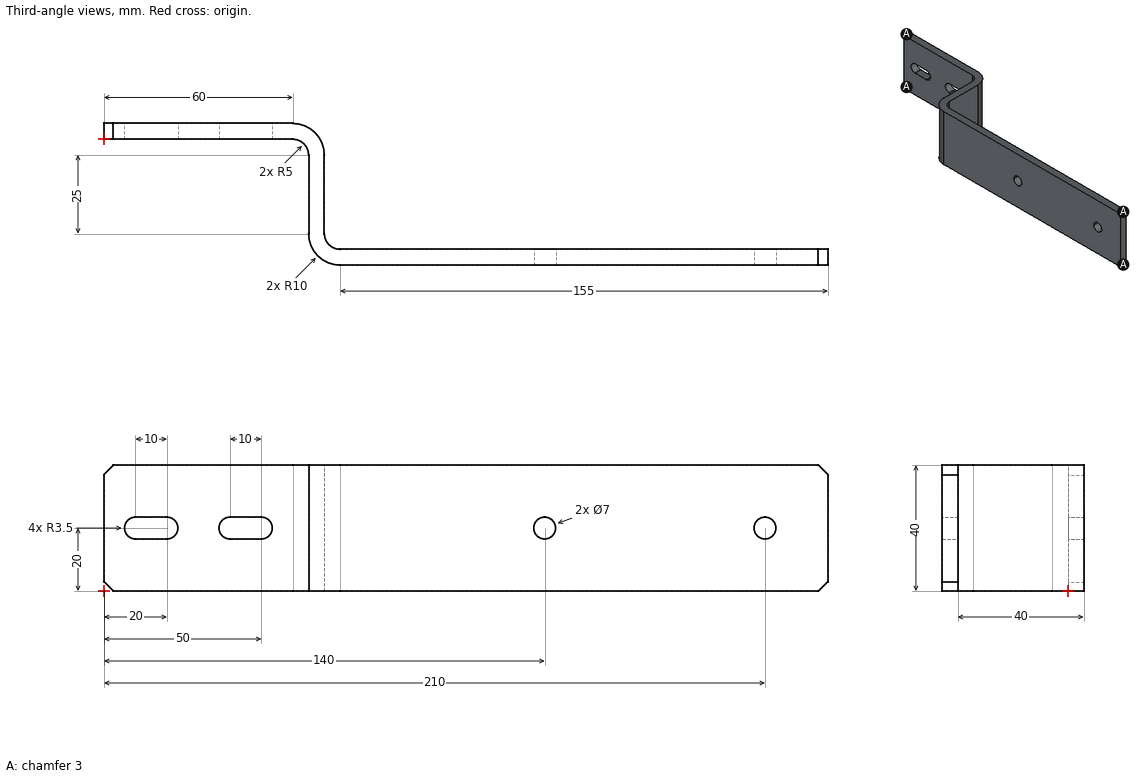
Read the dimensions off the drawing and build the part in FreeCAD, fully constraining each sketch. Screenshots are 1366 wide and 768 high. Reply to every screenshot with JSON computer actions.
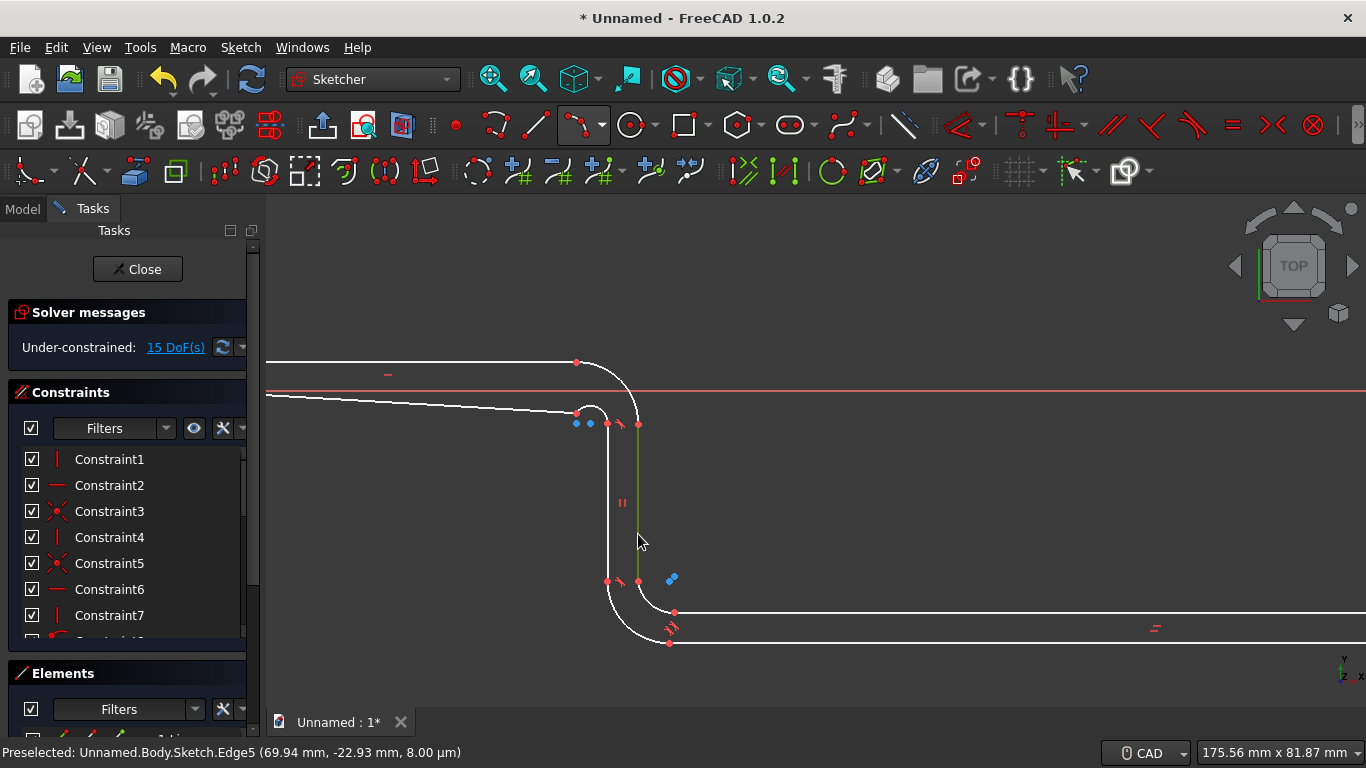
{"action": "left_click", "coordinate": [644, 596]}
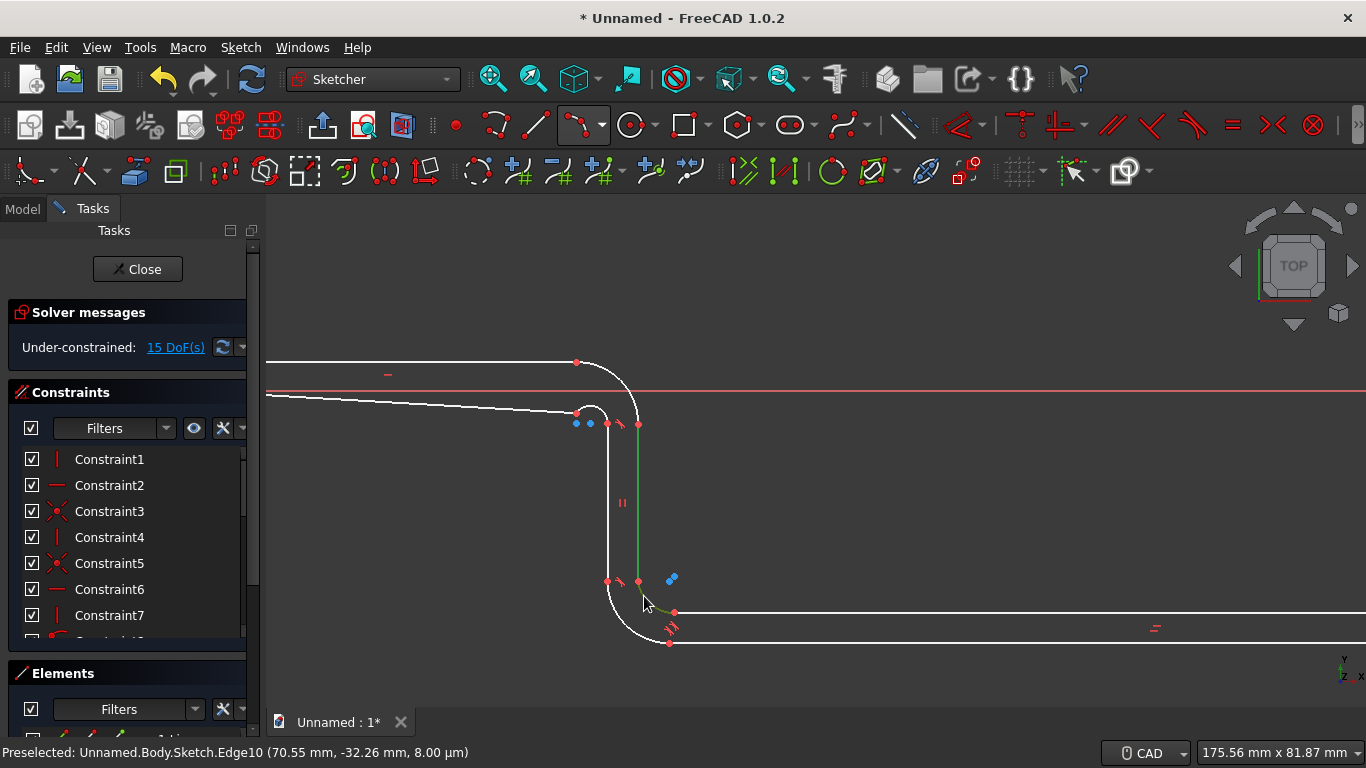
{"action": "left_click", "coordinate": [1194, 126]}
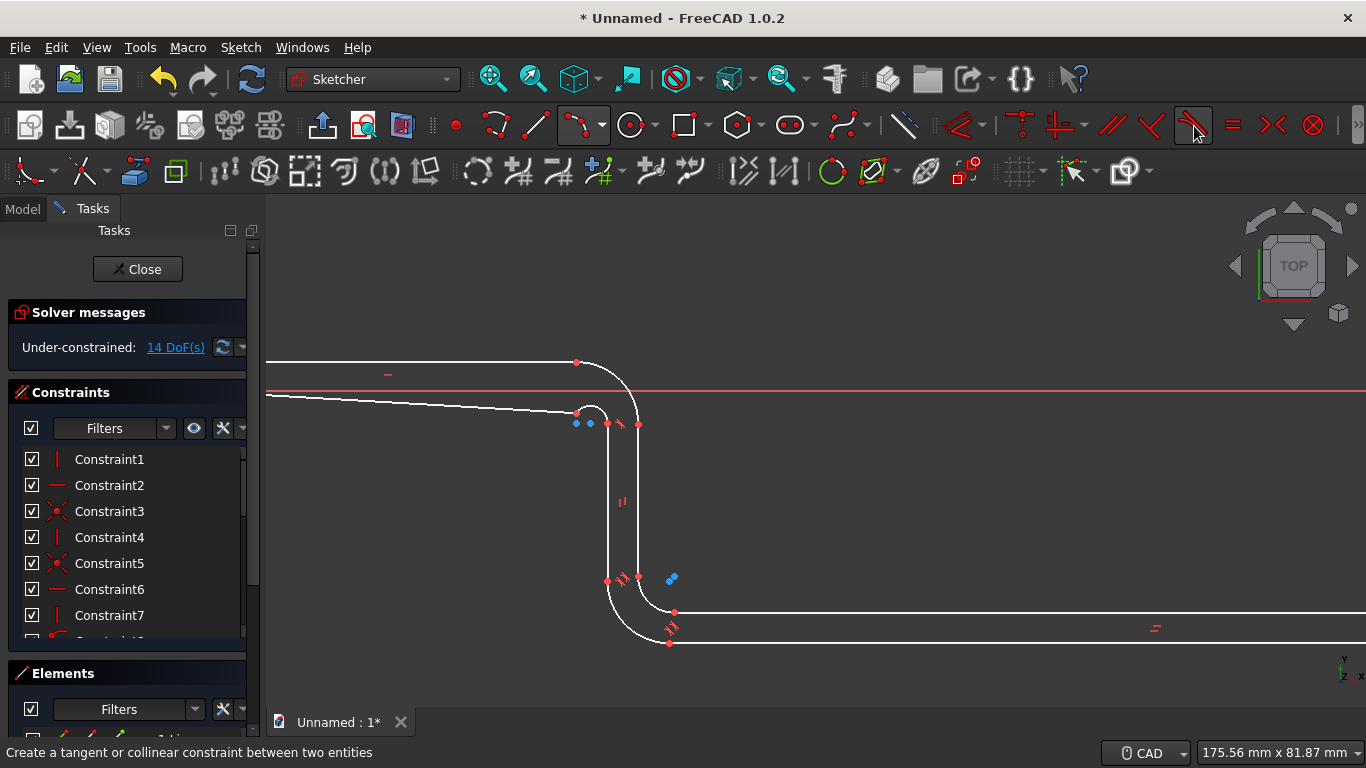
{"action": "left_click", "coordinate": [638, 531]}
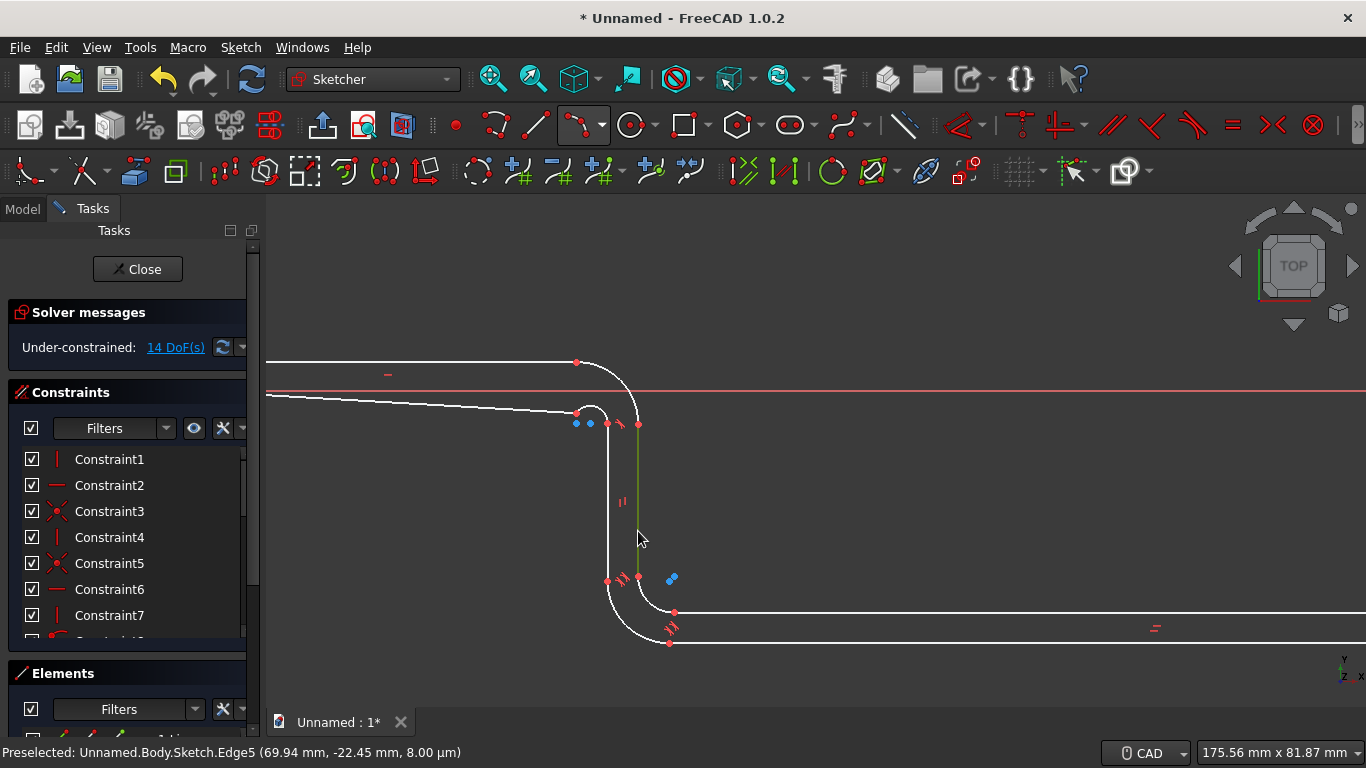
{"action": "left_click", "coordinate": [604, 369]}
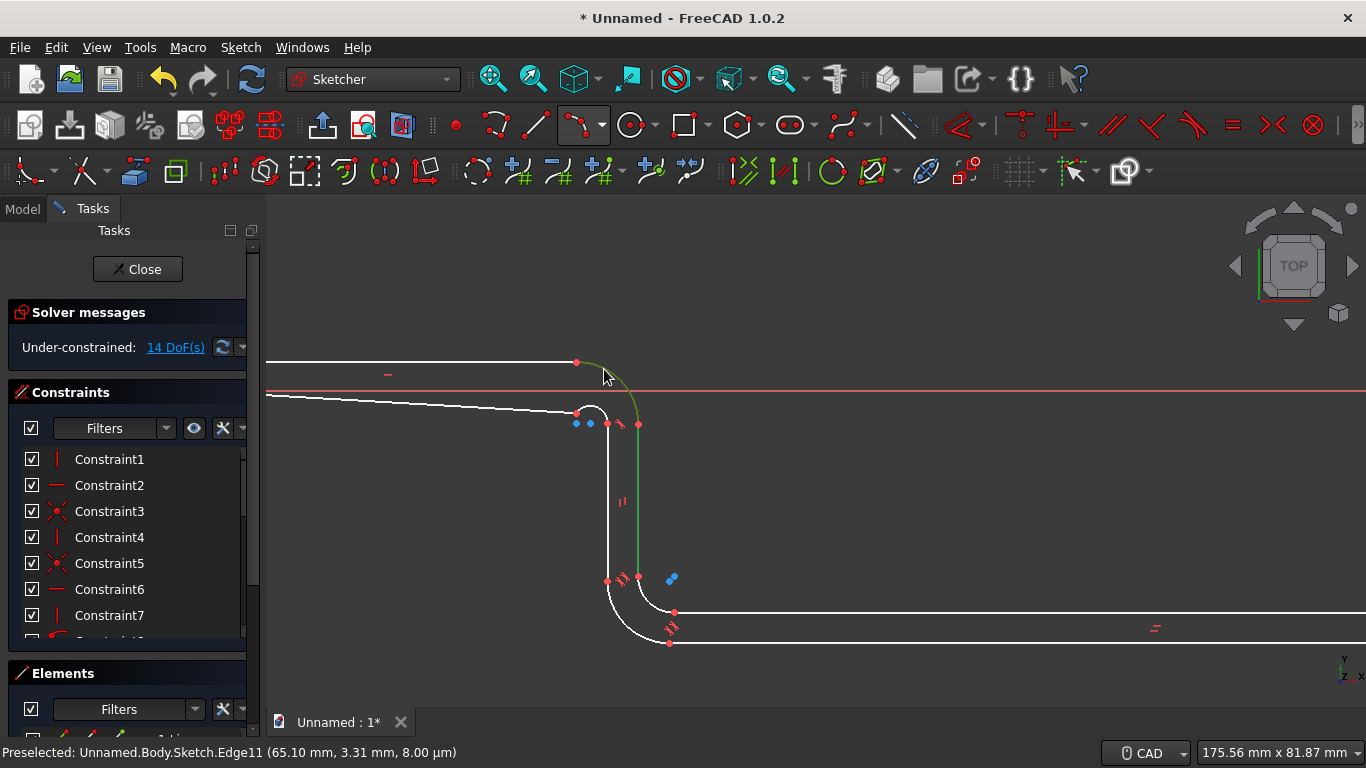
{"action": "left_click", "coordinate": [1194, 126]}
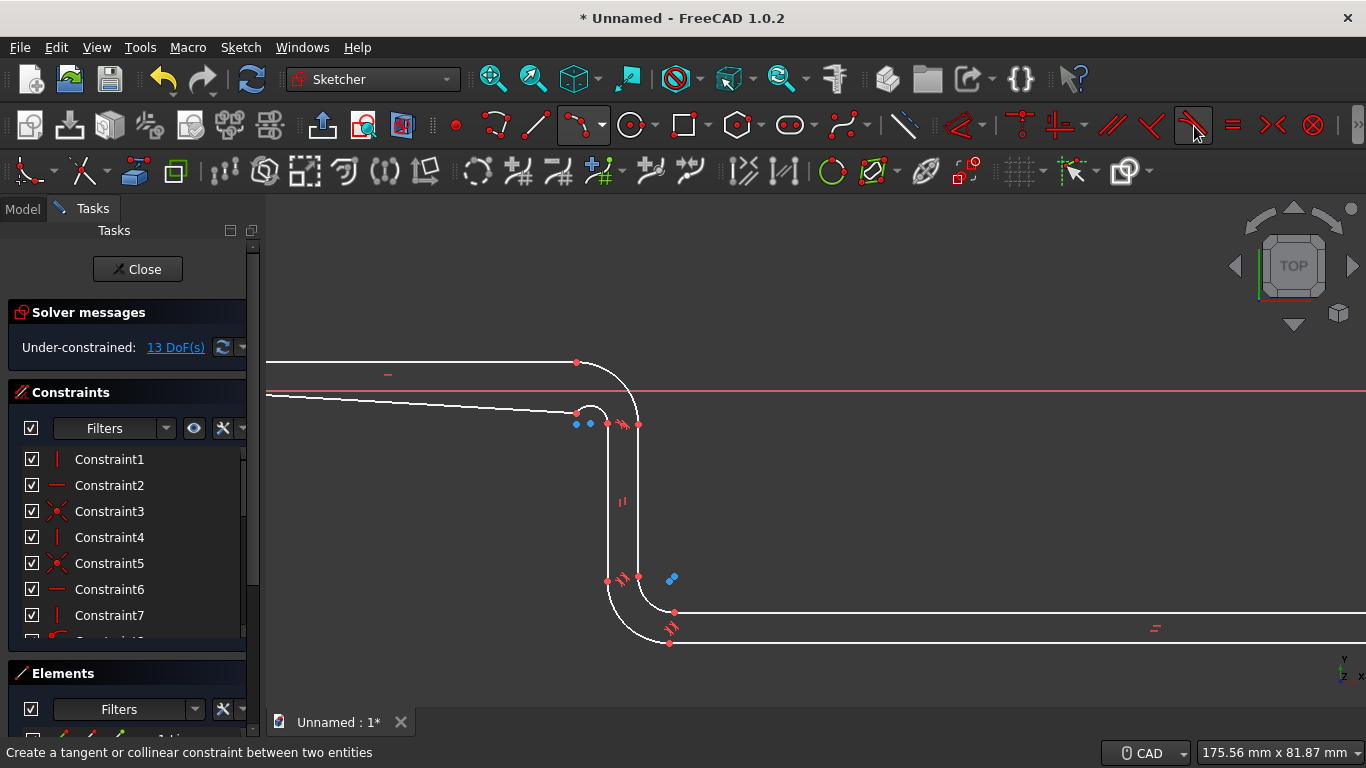
{"action": "left_click", "coordinate": [463, 362]}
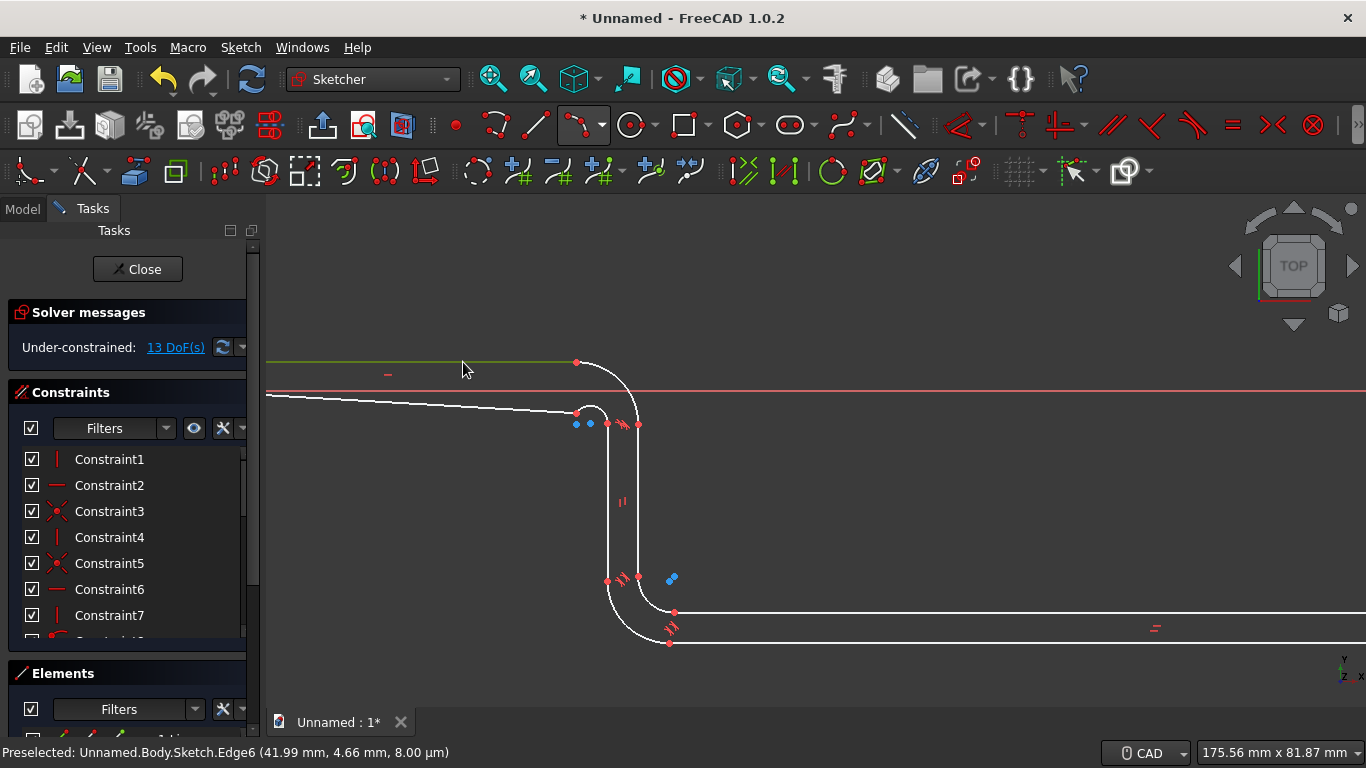
{"action": "left_click", "coordinate": [604, 369]}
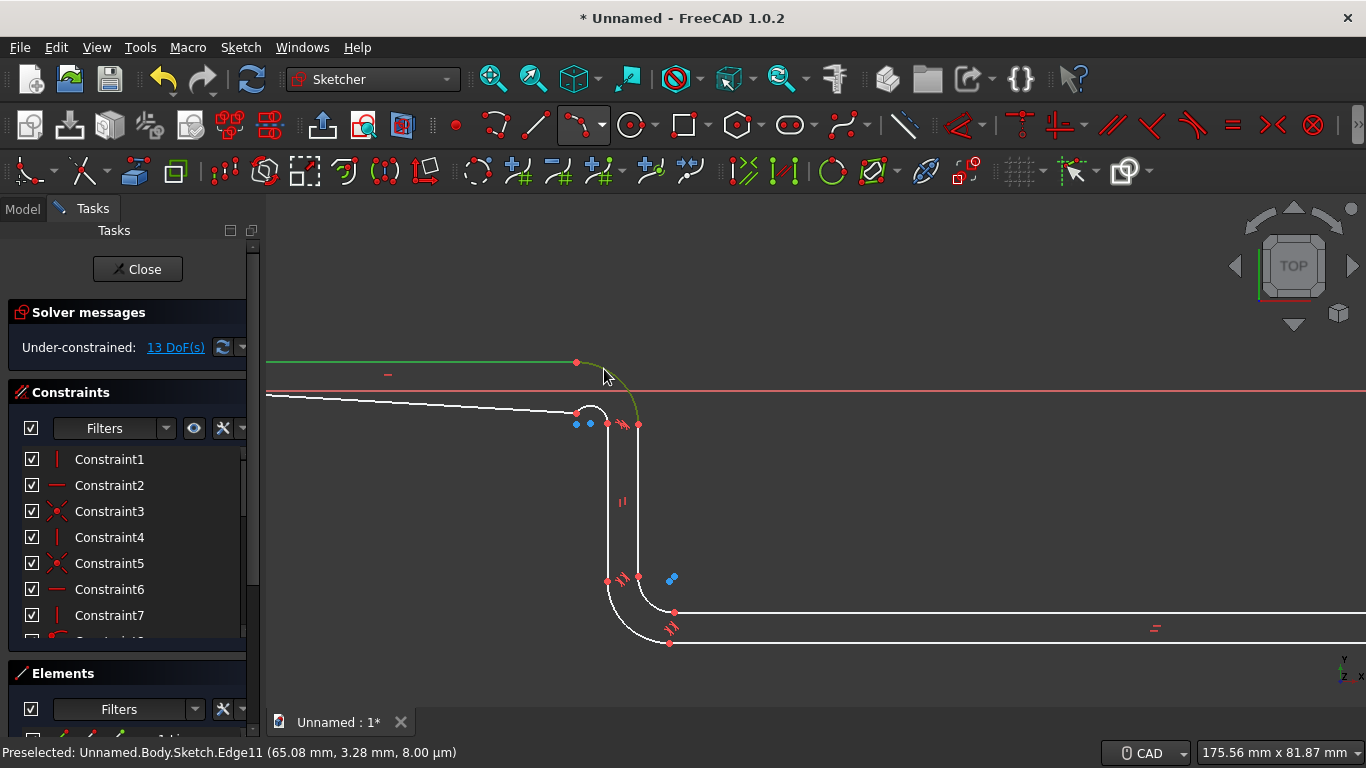
{"action": "left_click", "coordinate": [1194, 126]}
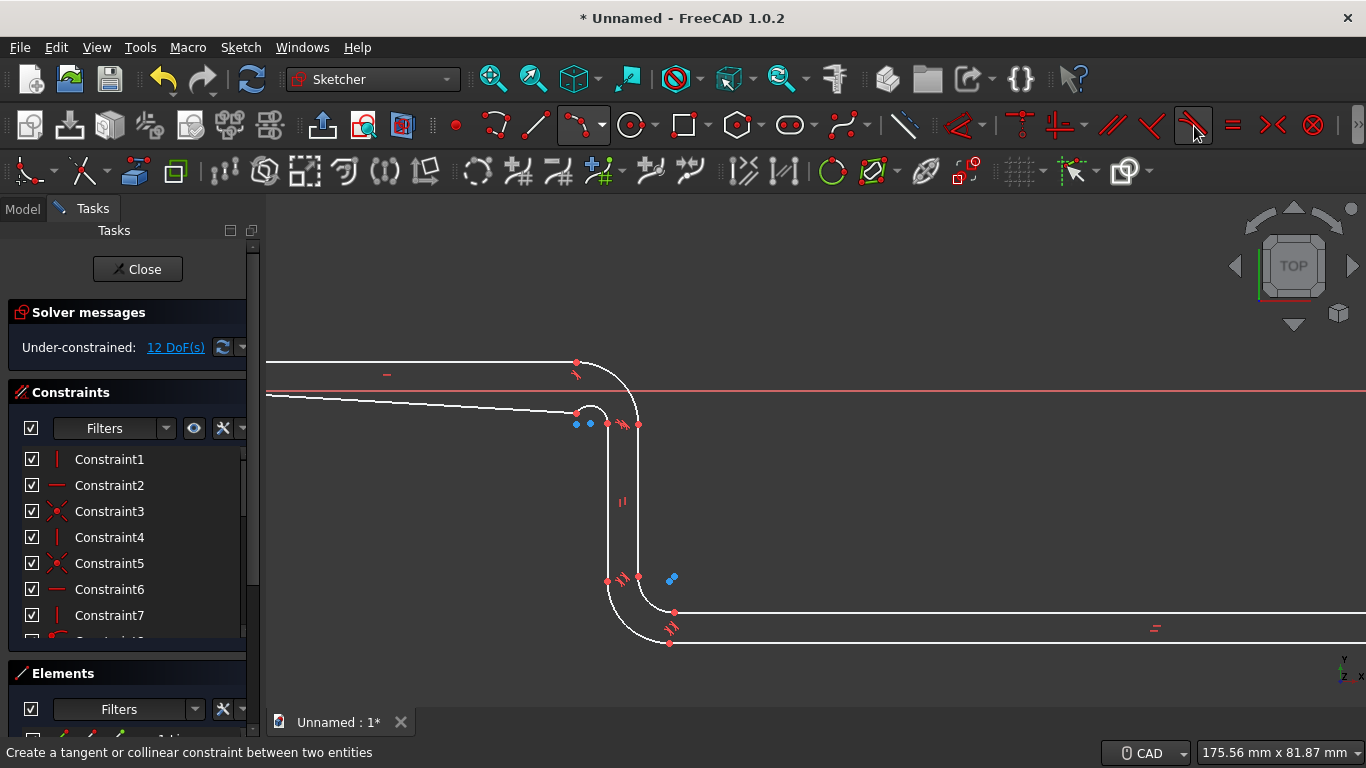
{"action": "left_click", "coordinate": [463, 407]}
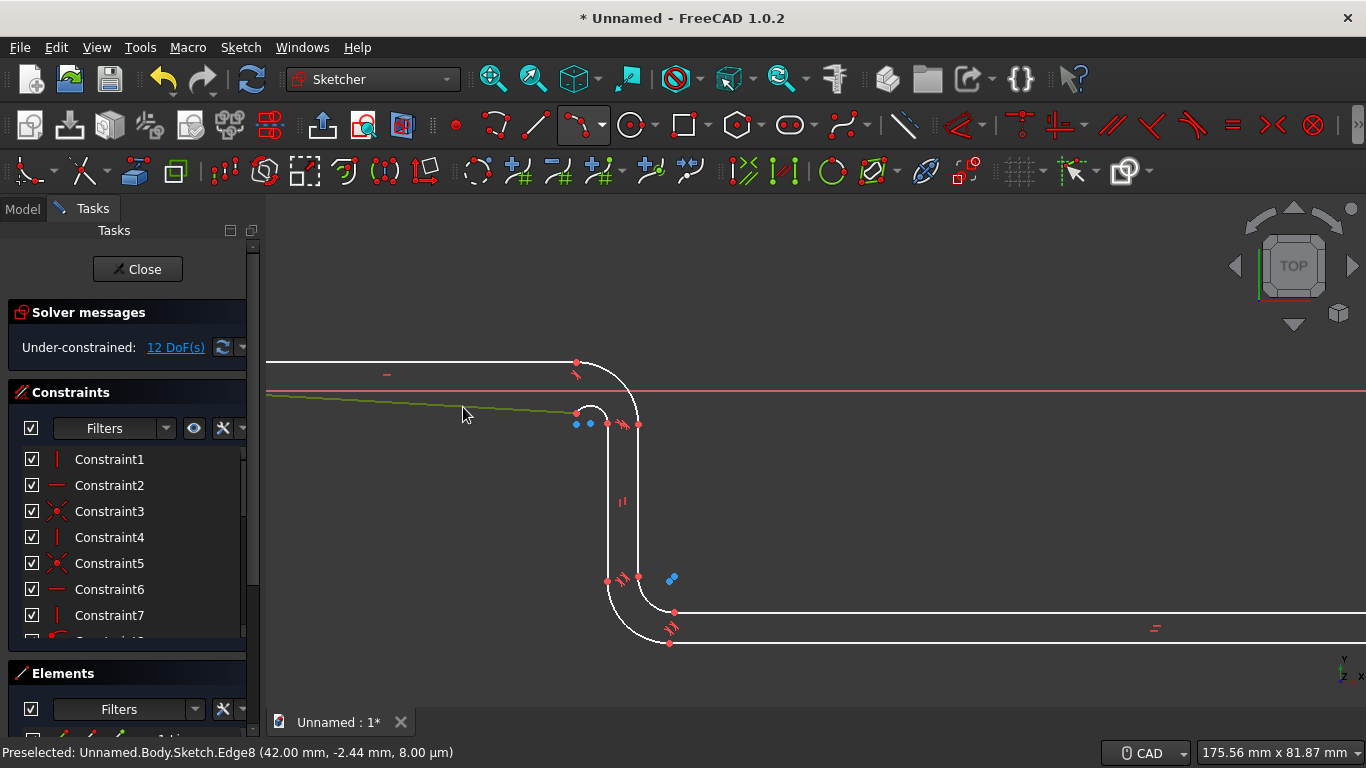
{"action": "left_click", "coordinate": [603, 411]}